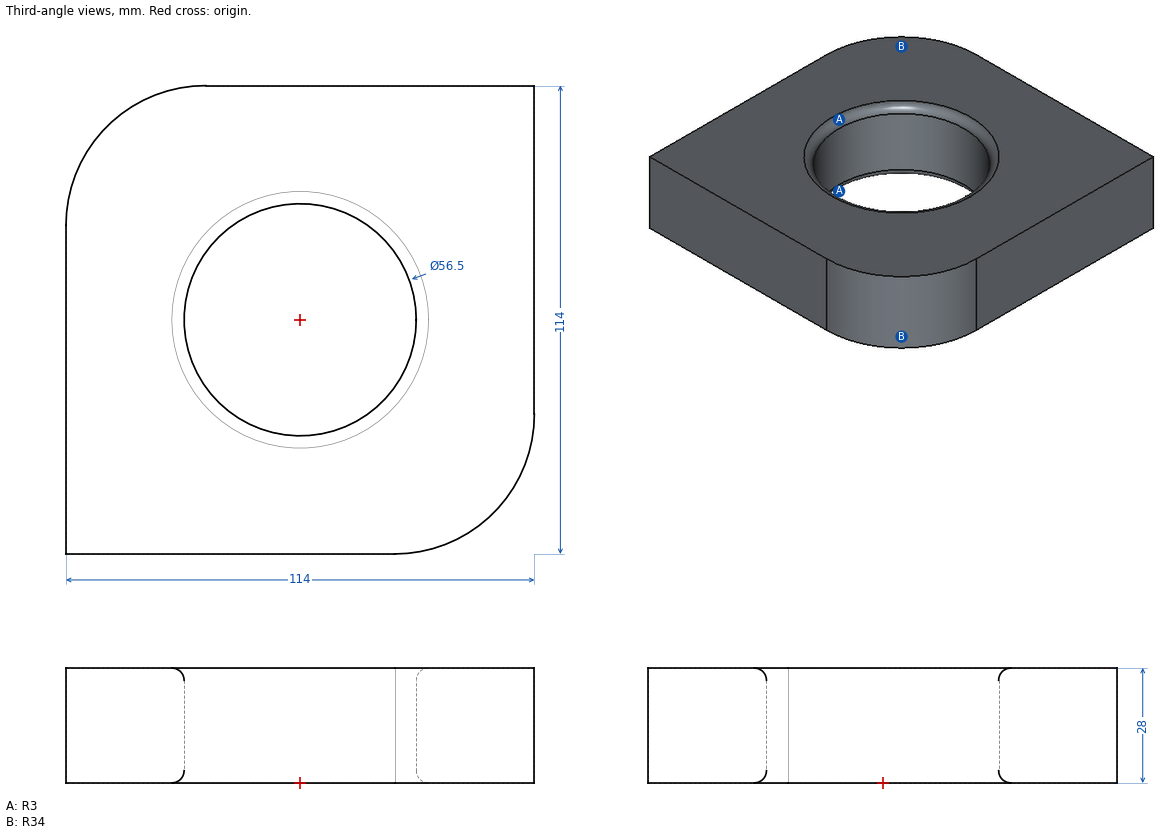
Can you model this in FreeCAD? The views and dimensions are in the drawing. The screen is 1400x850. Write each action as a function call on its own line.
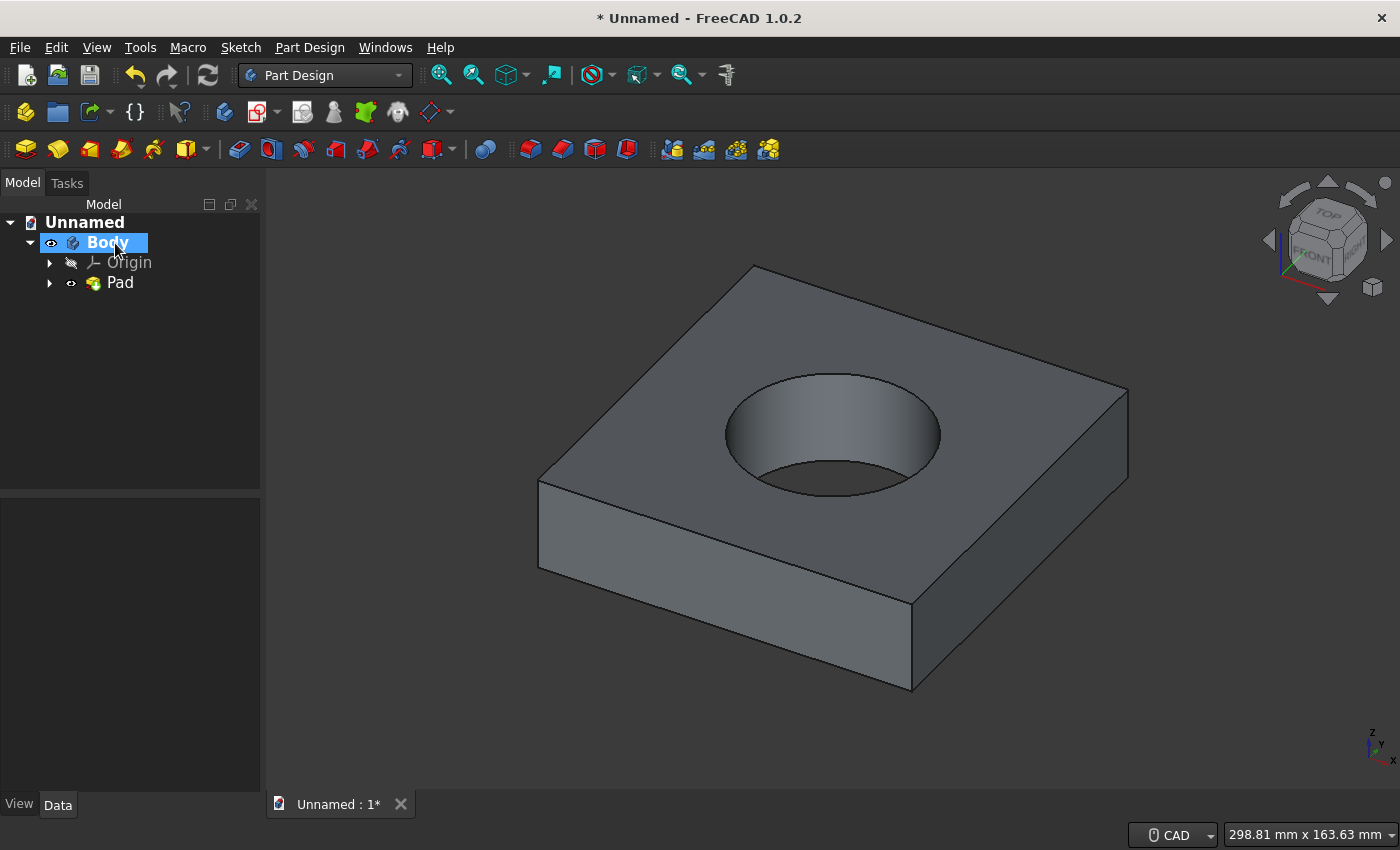
click(740, 403)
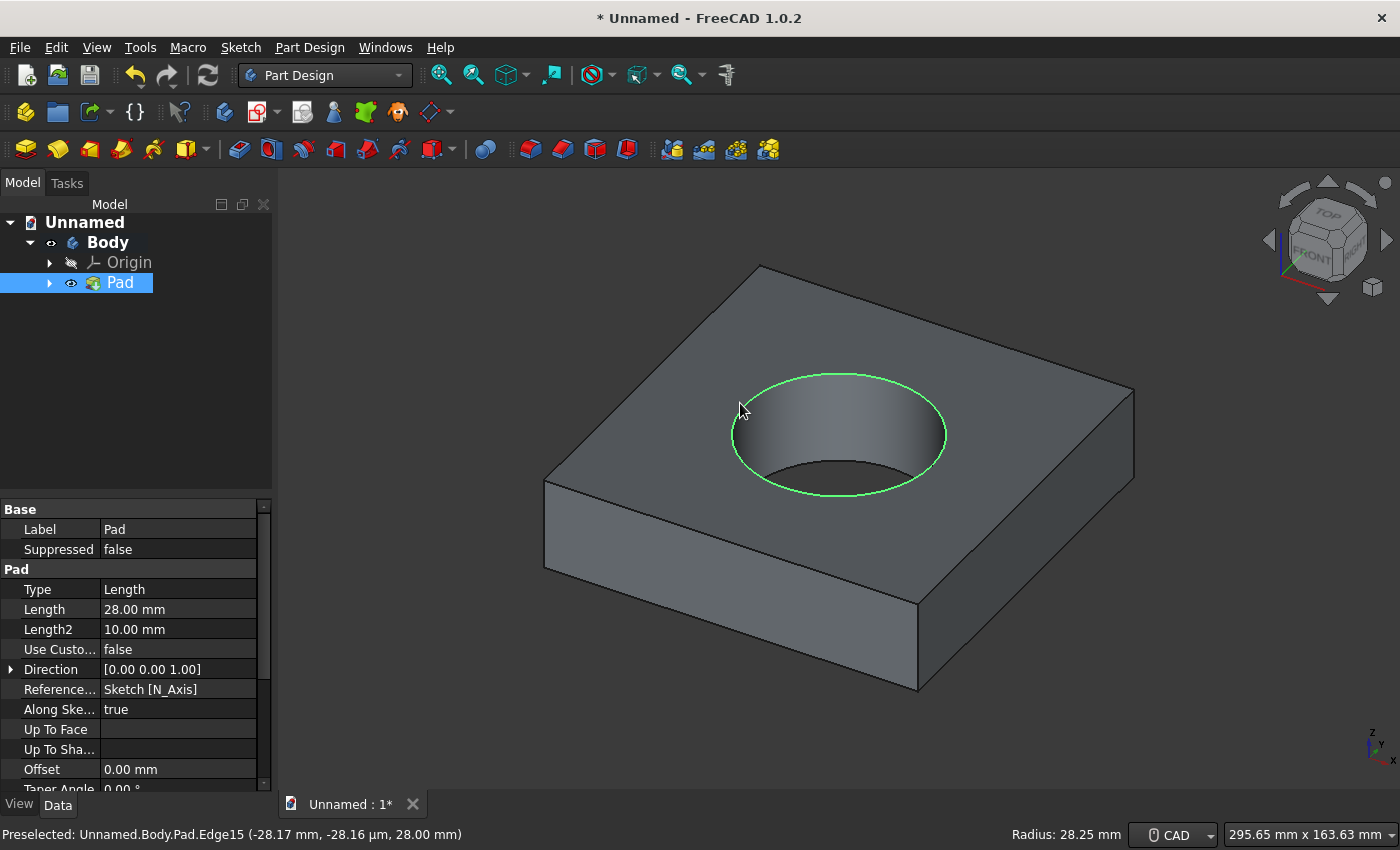
key(0)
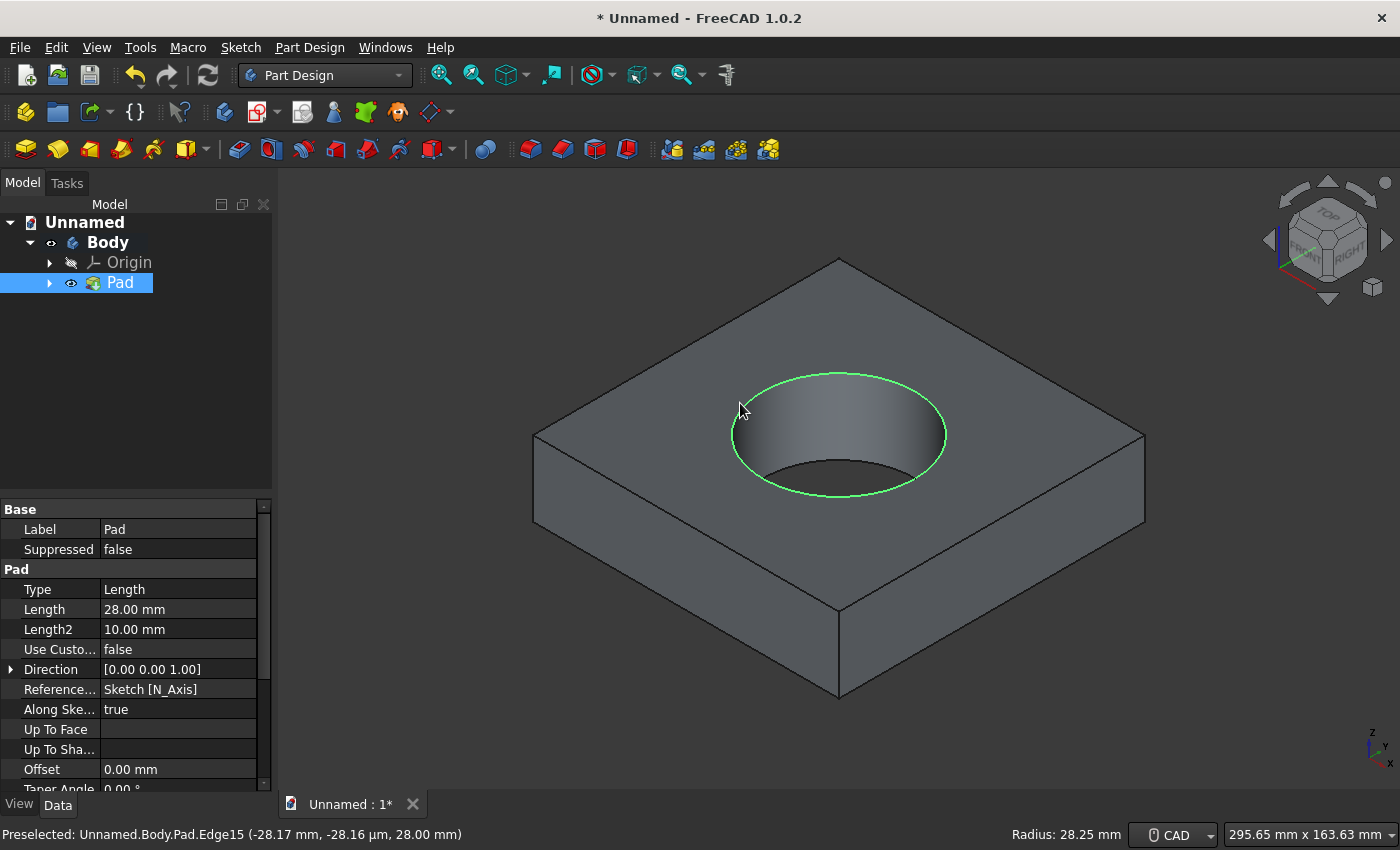
key(2)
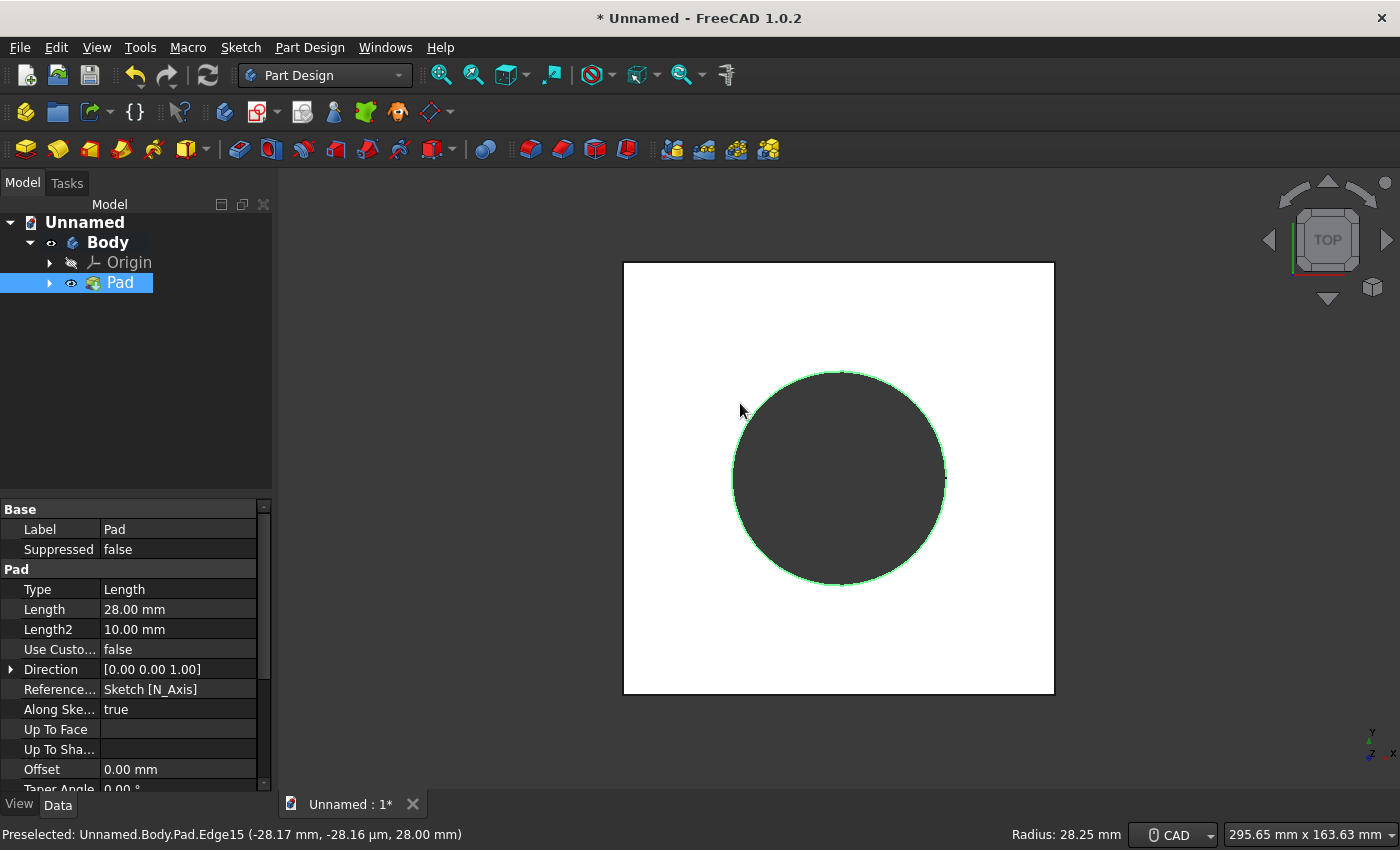
key(1)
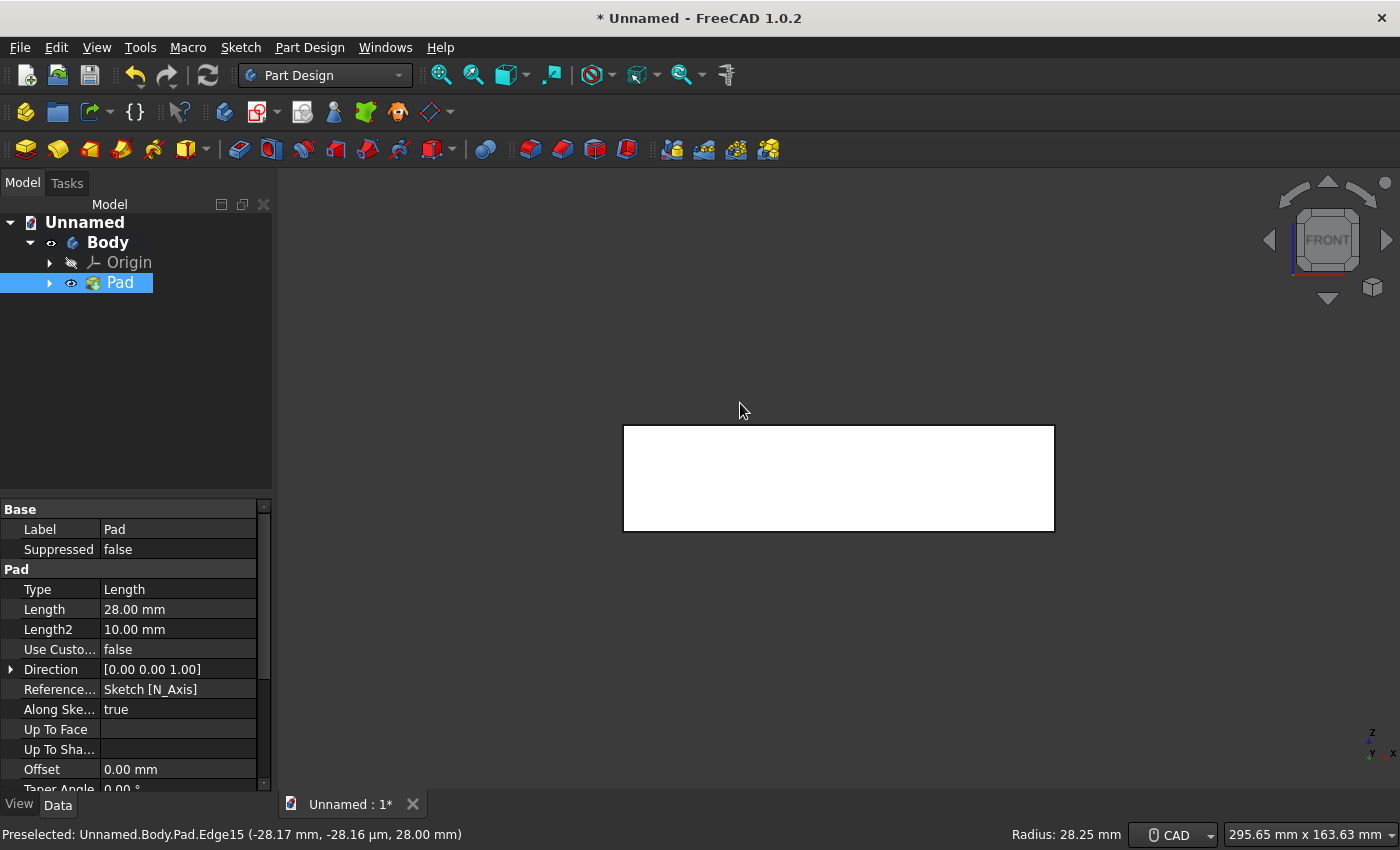
click(442, 76)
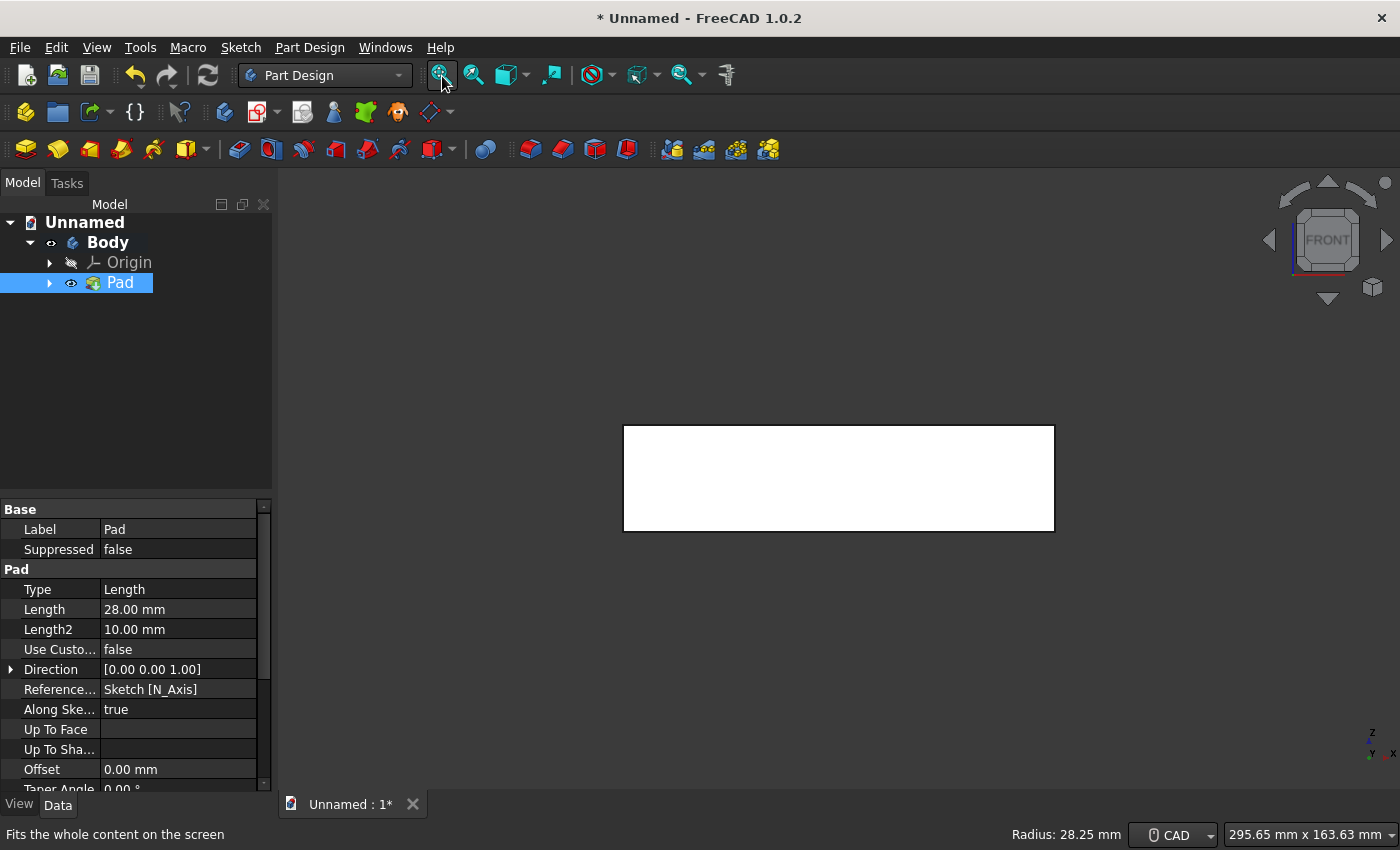
key(3)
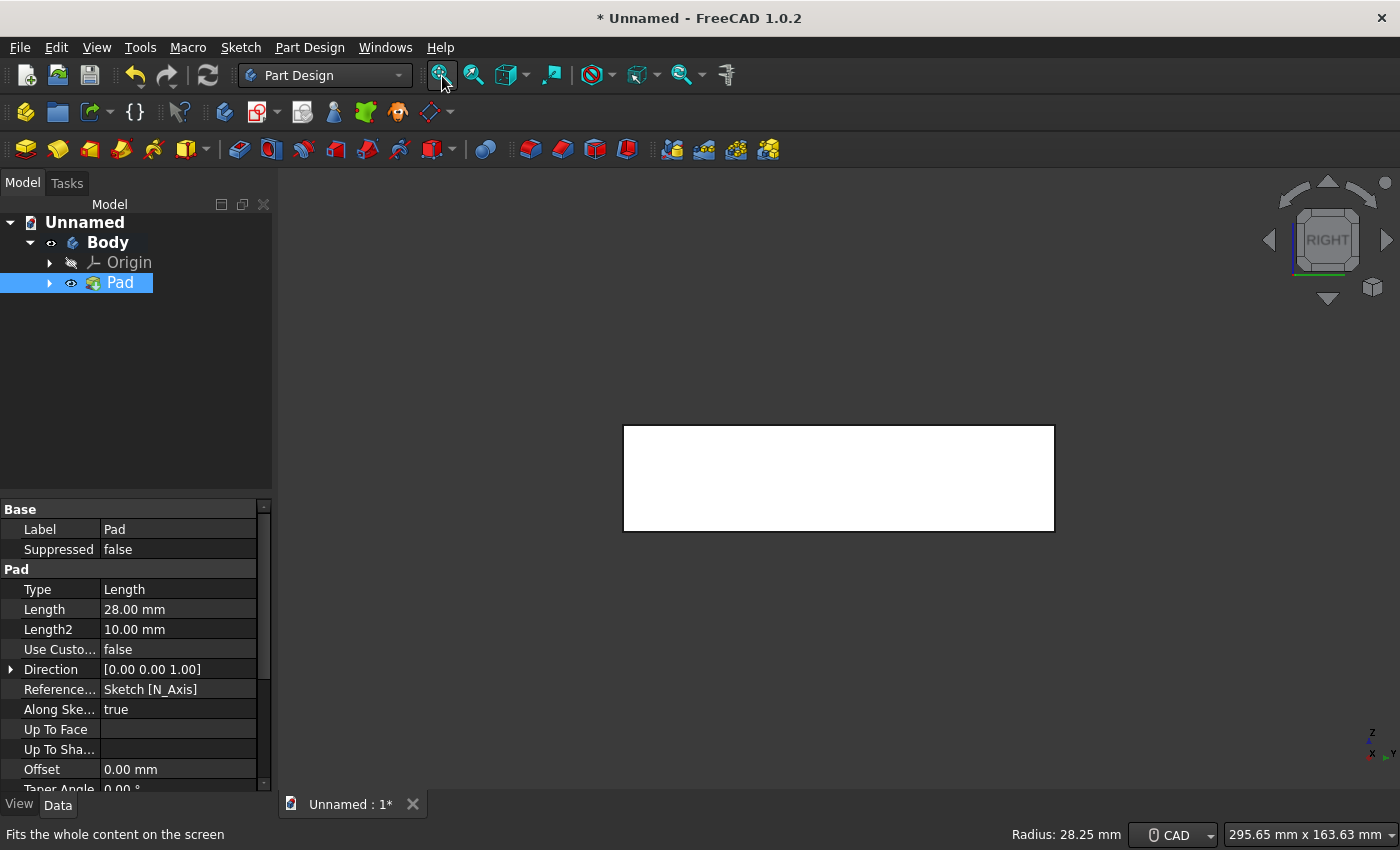
key(v)
key(f)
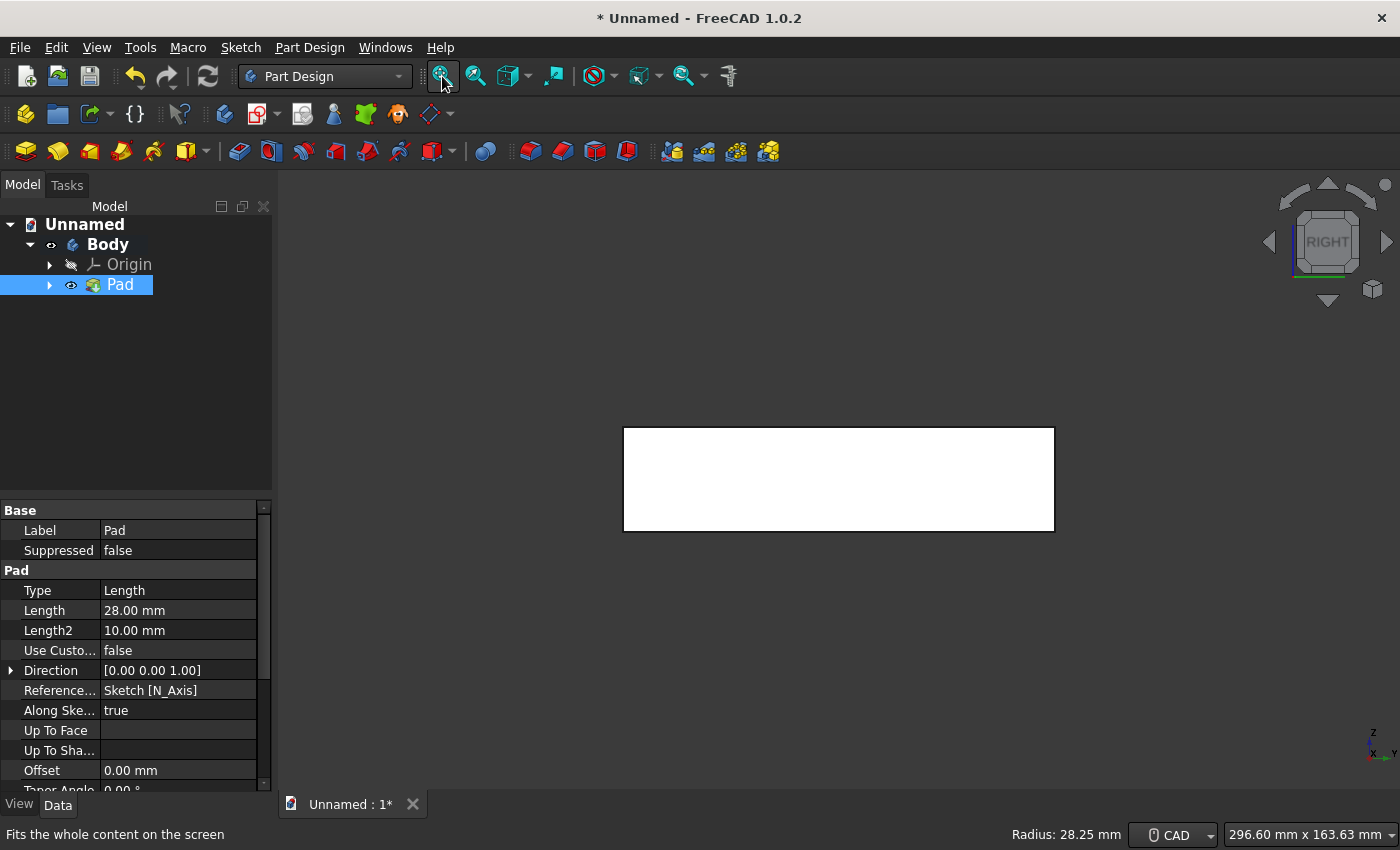
key(5)